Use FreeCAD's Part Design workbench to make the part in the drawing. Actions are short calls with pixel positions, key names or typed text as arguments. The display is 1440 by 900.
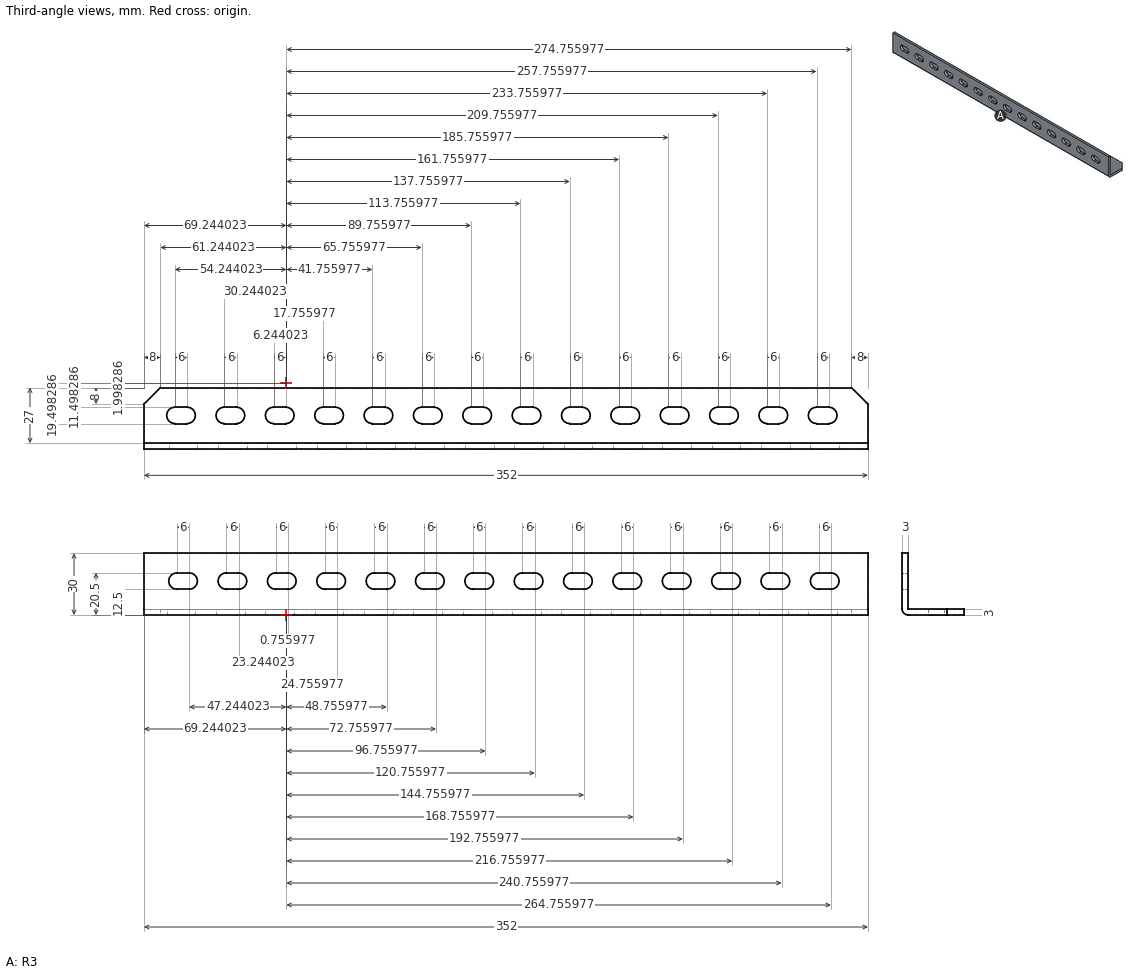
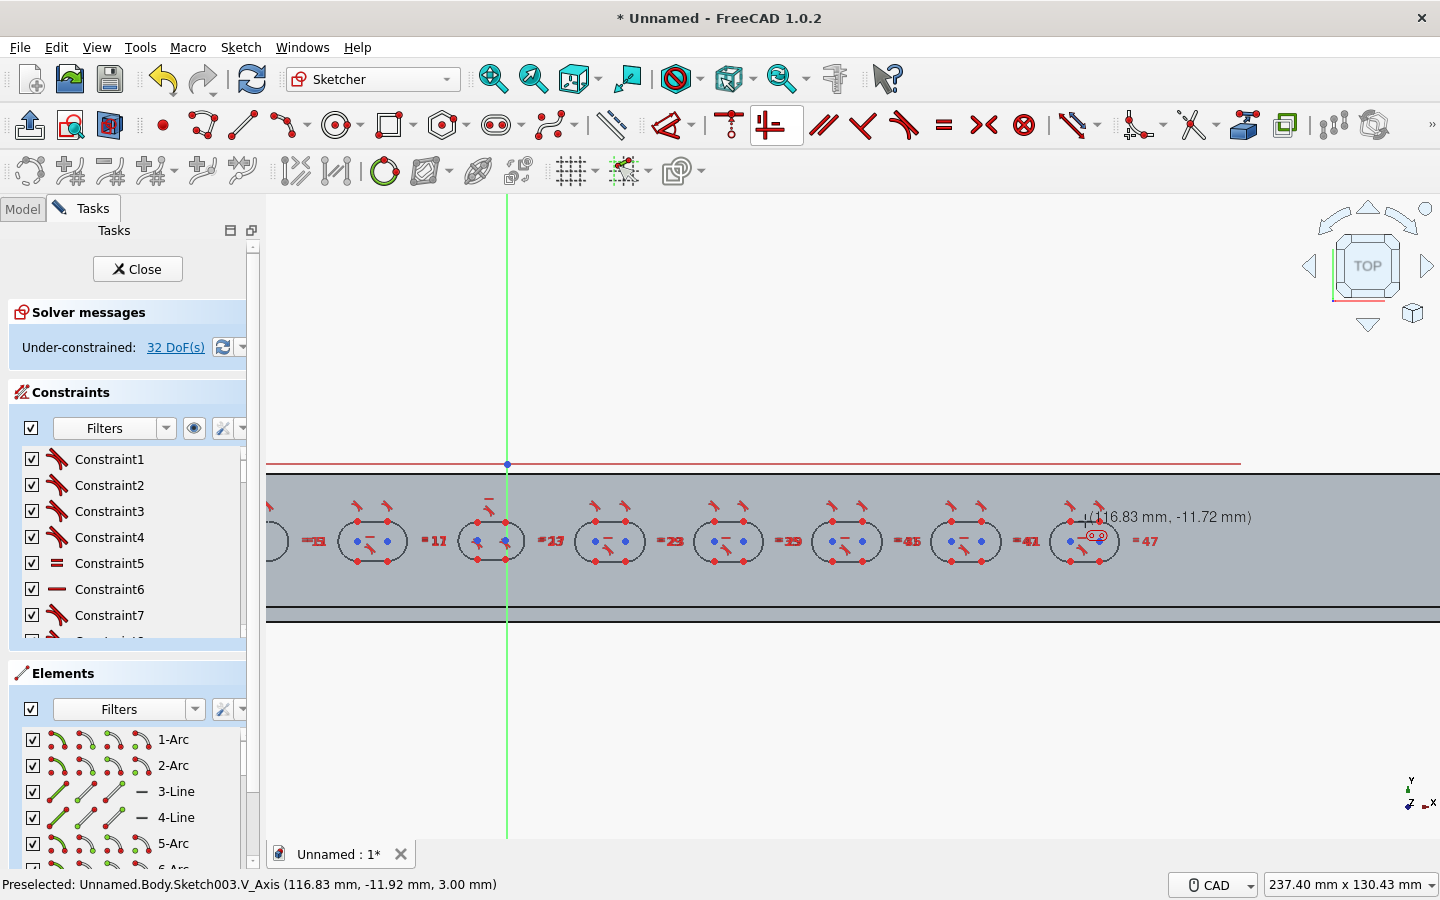
click(1189, 541)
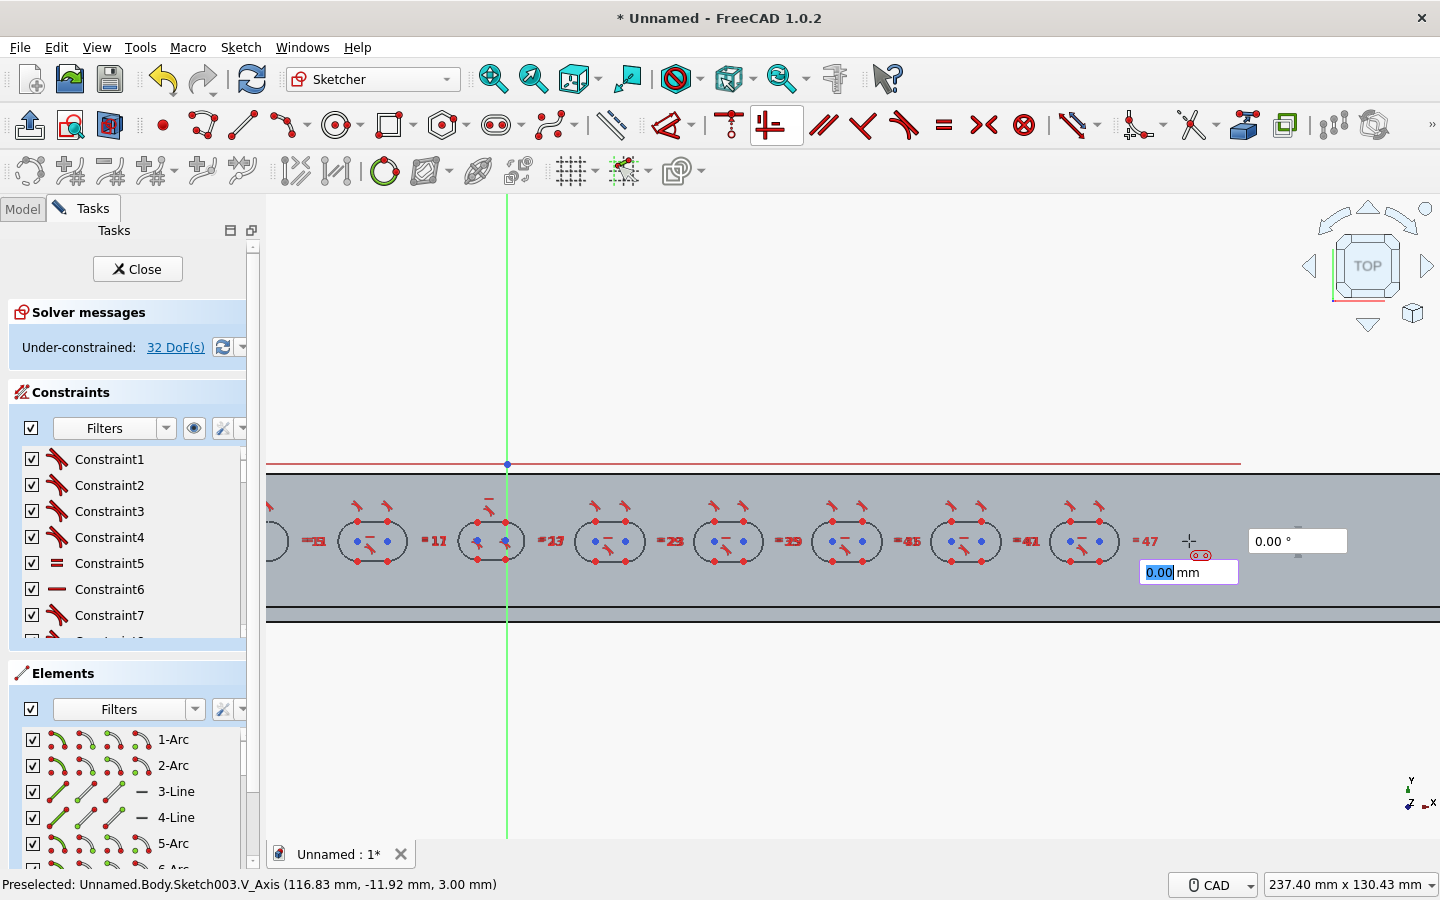
click(1218, 541)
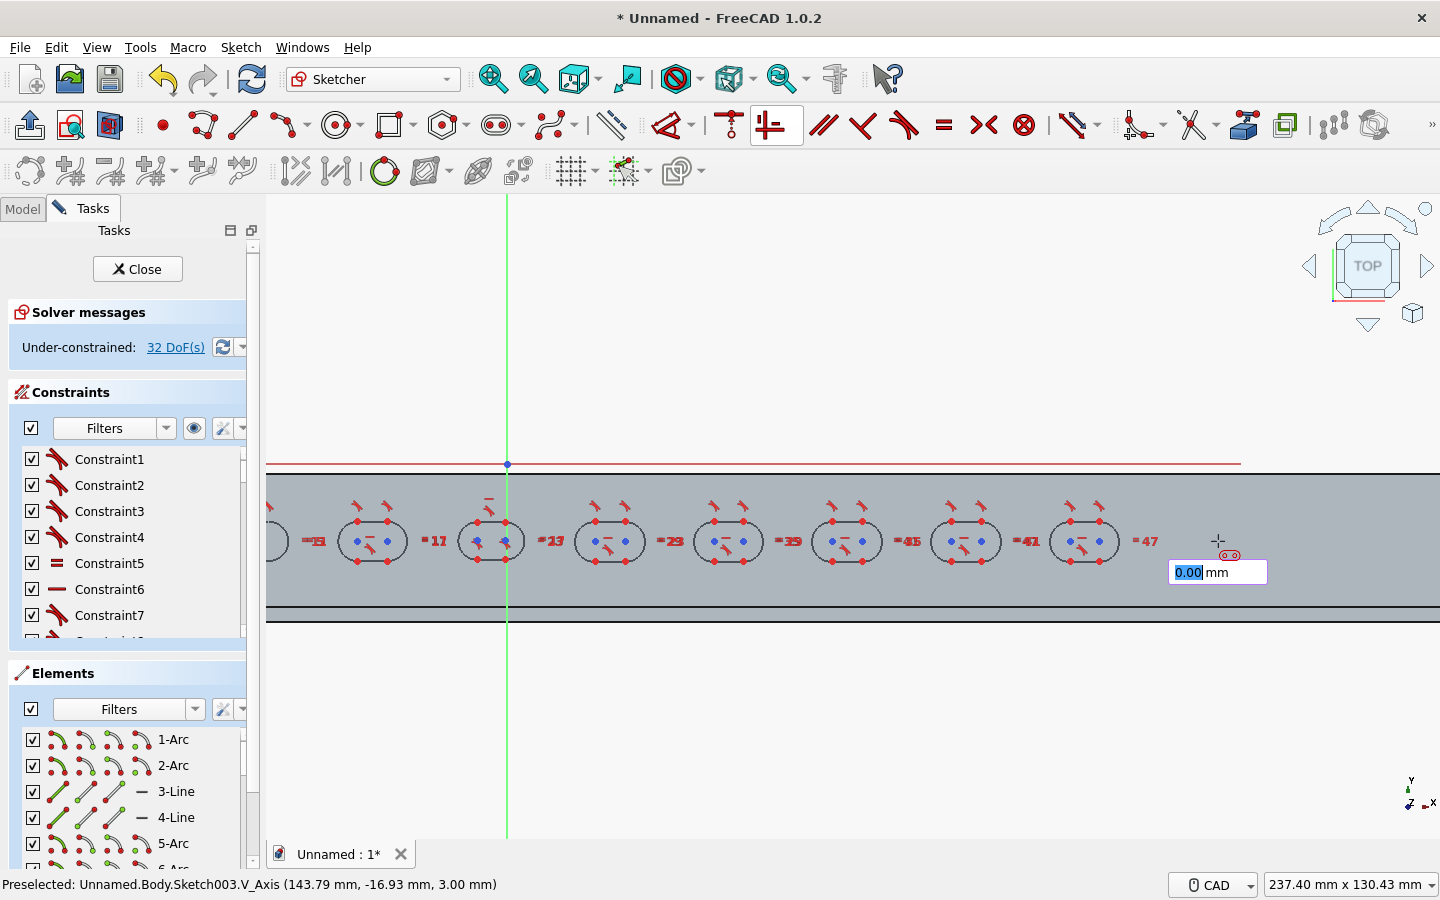
click(1203, 521)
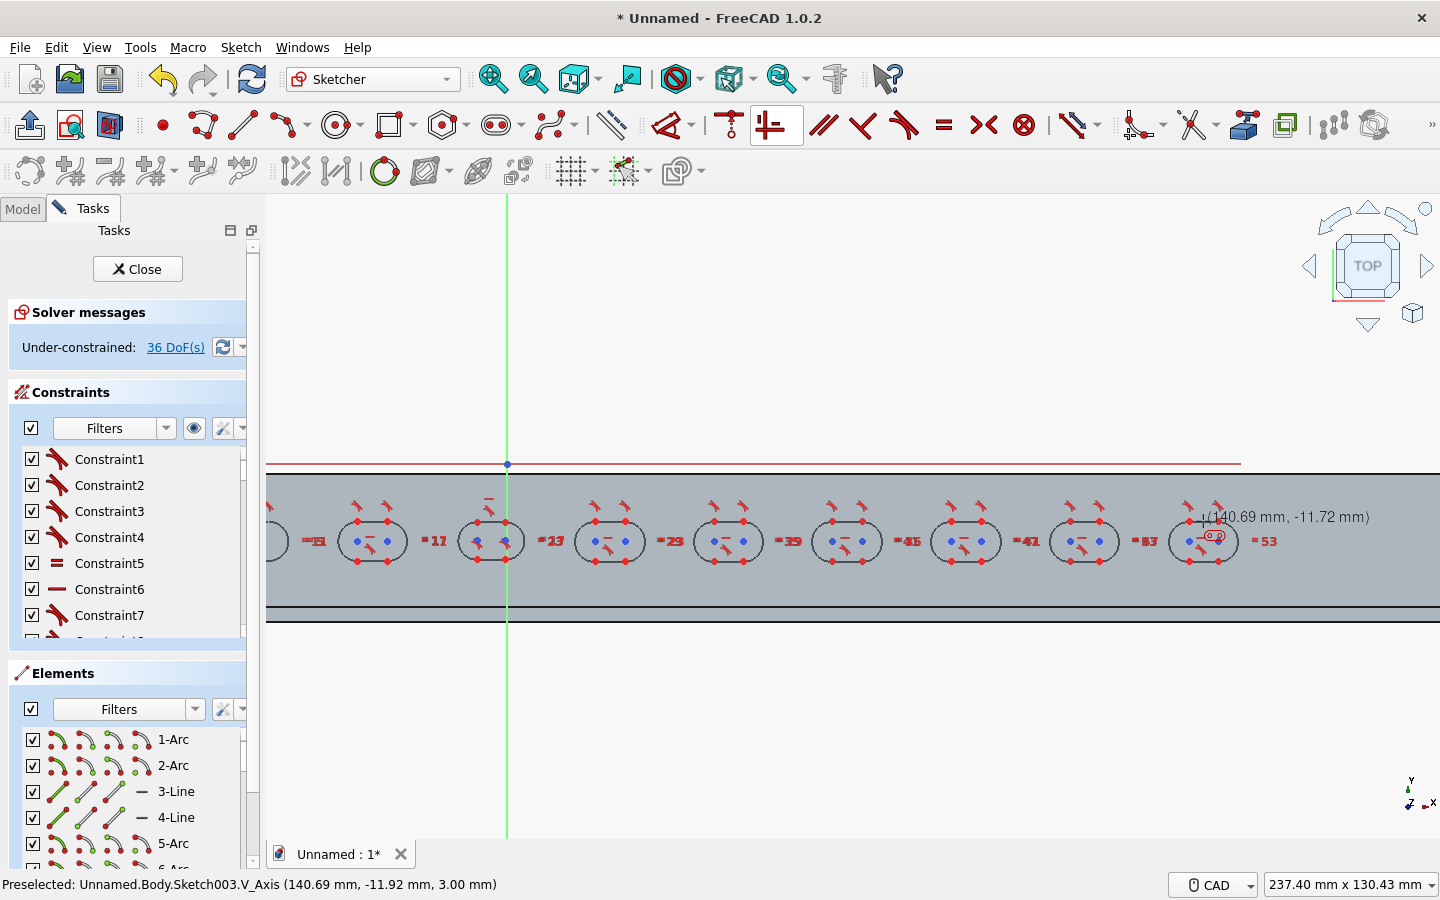
scroll(588, 520, down, 4)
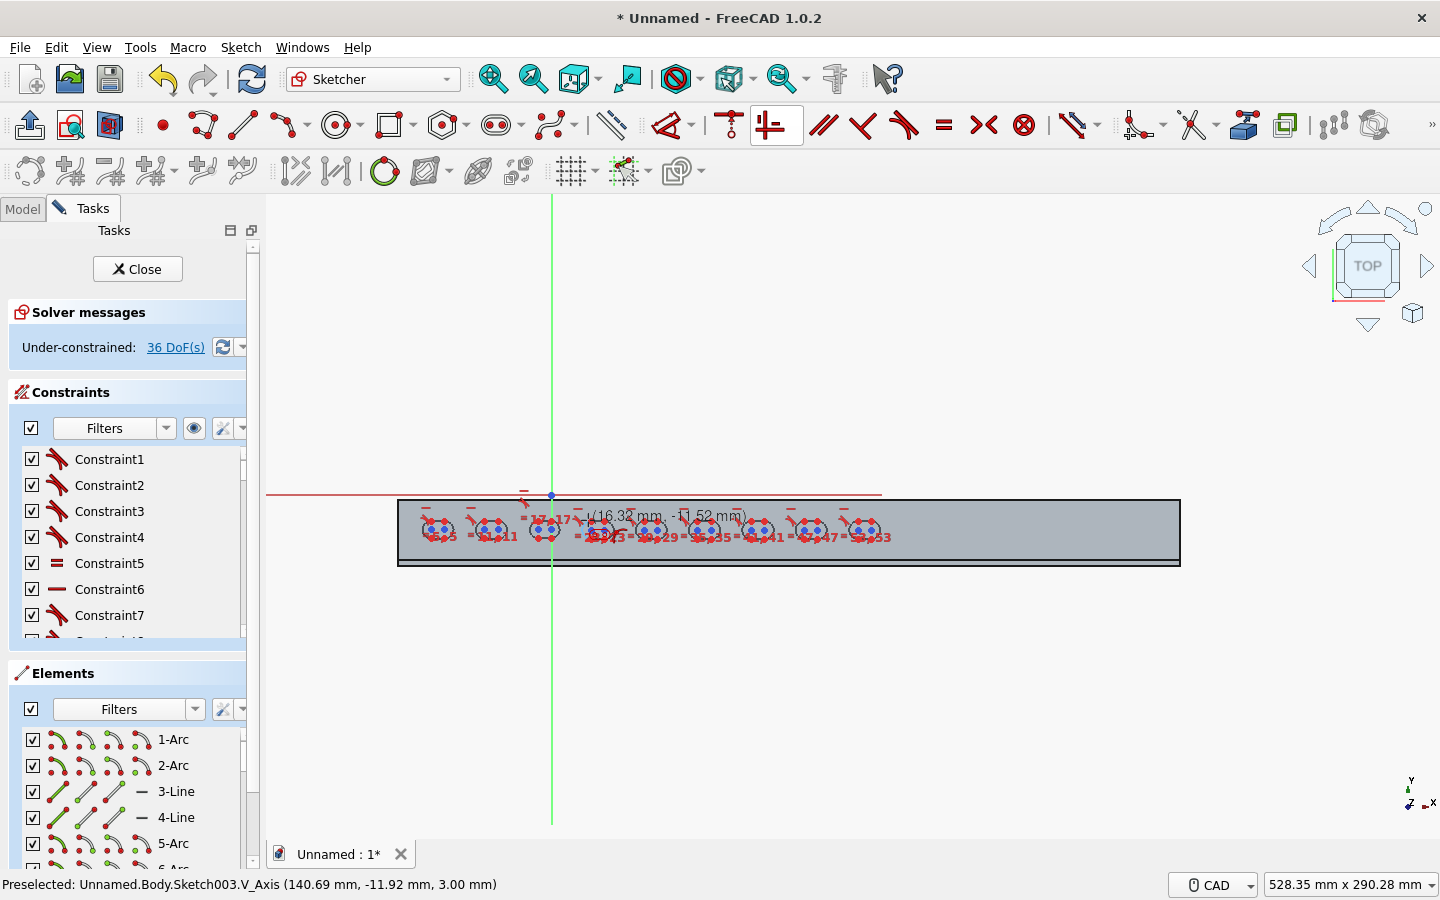
scroll(911, 530, up, 5)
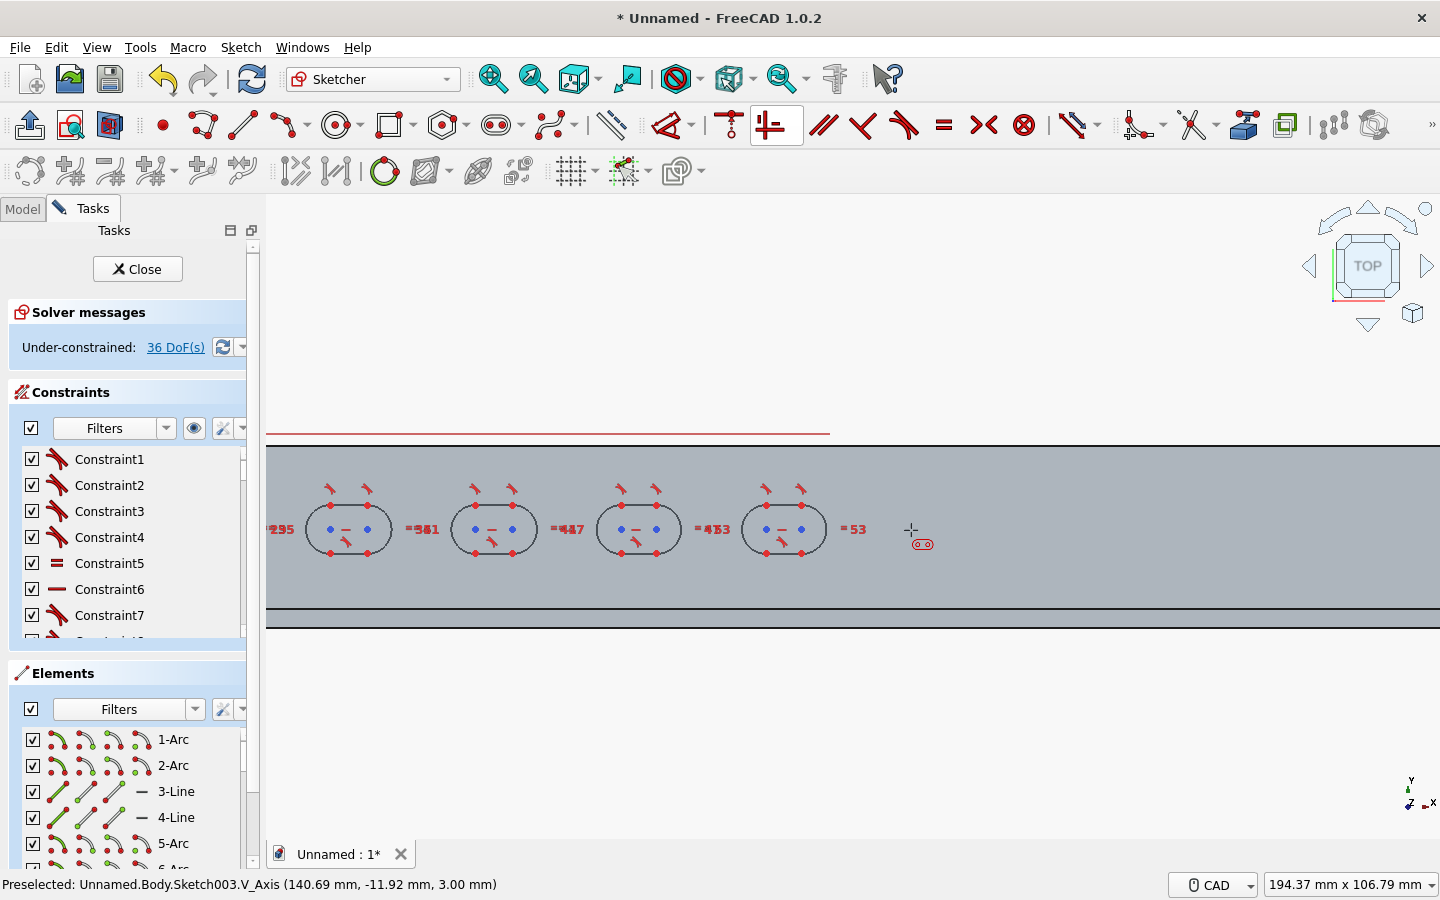
click(911, 528)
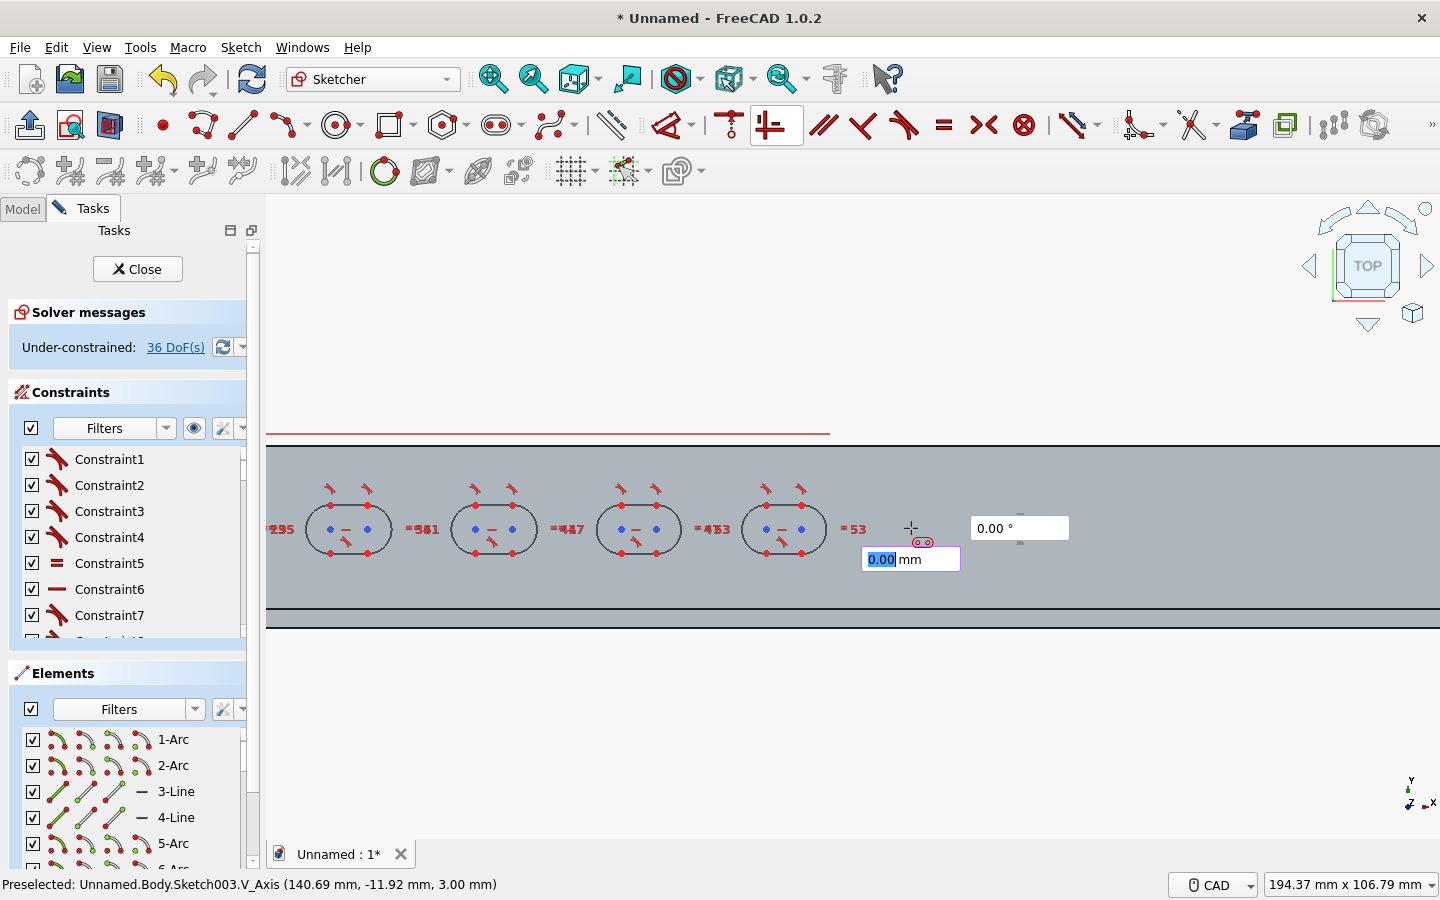
click(947, 528)